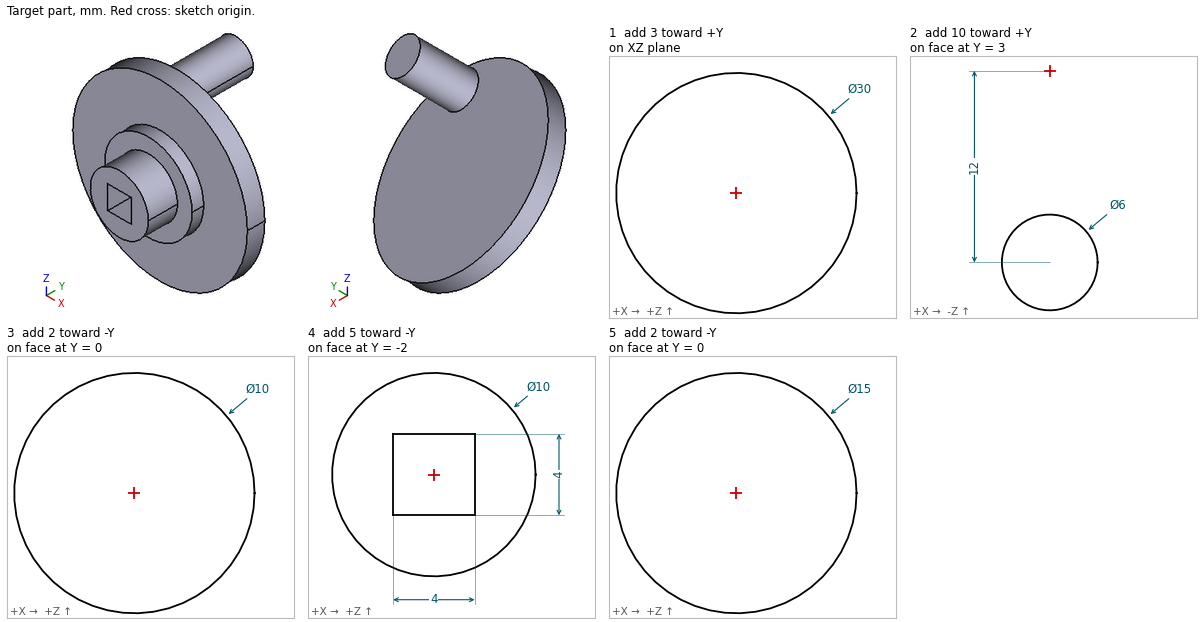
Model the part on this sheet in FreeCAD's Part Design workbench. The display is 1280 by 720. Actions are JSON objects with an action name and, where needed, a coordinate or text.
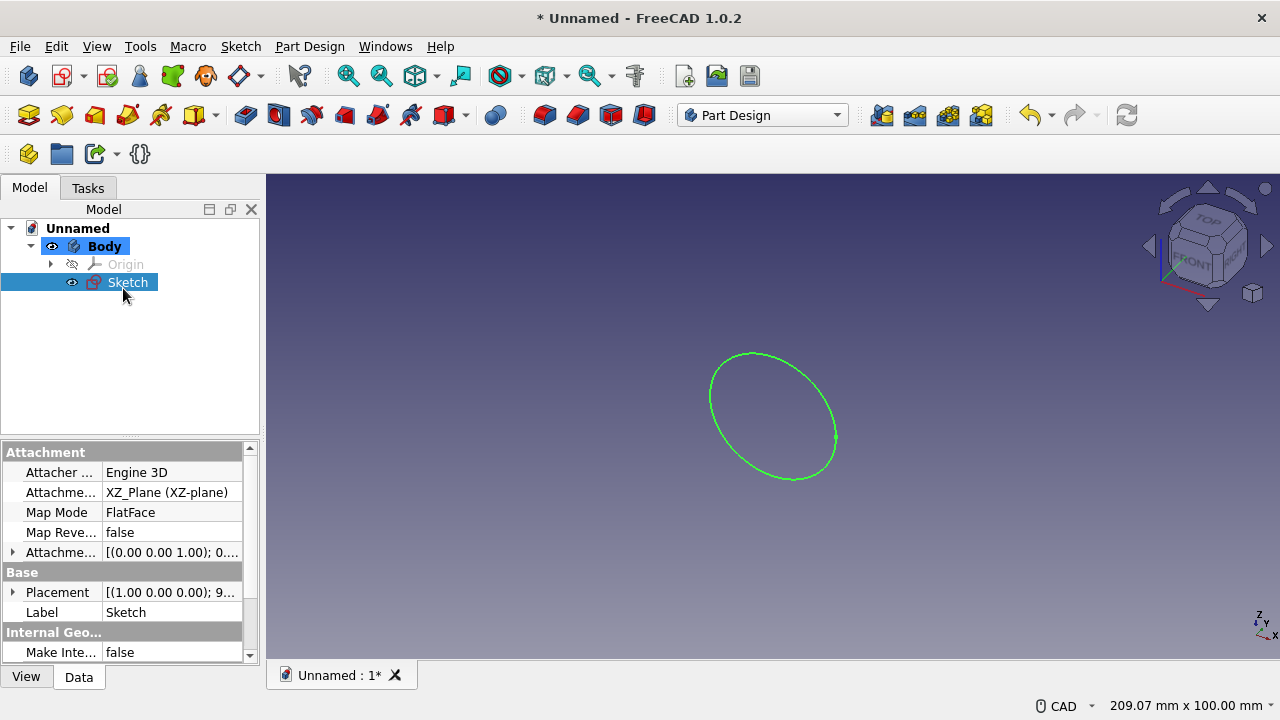
{"action": "left_click", "coordinate": [29, 116]}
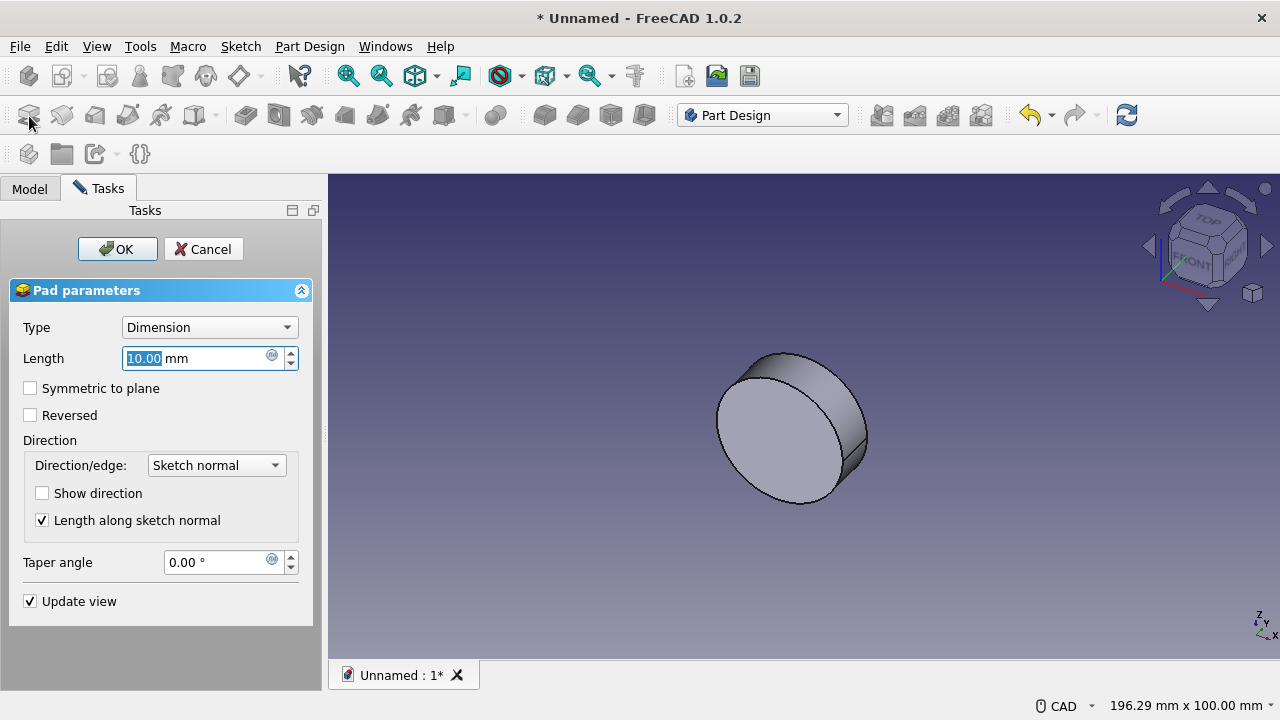
{"action": "type", "text": "3"}
{"action": "key", "text": "Tab"}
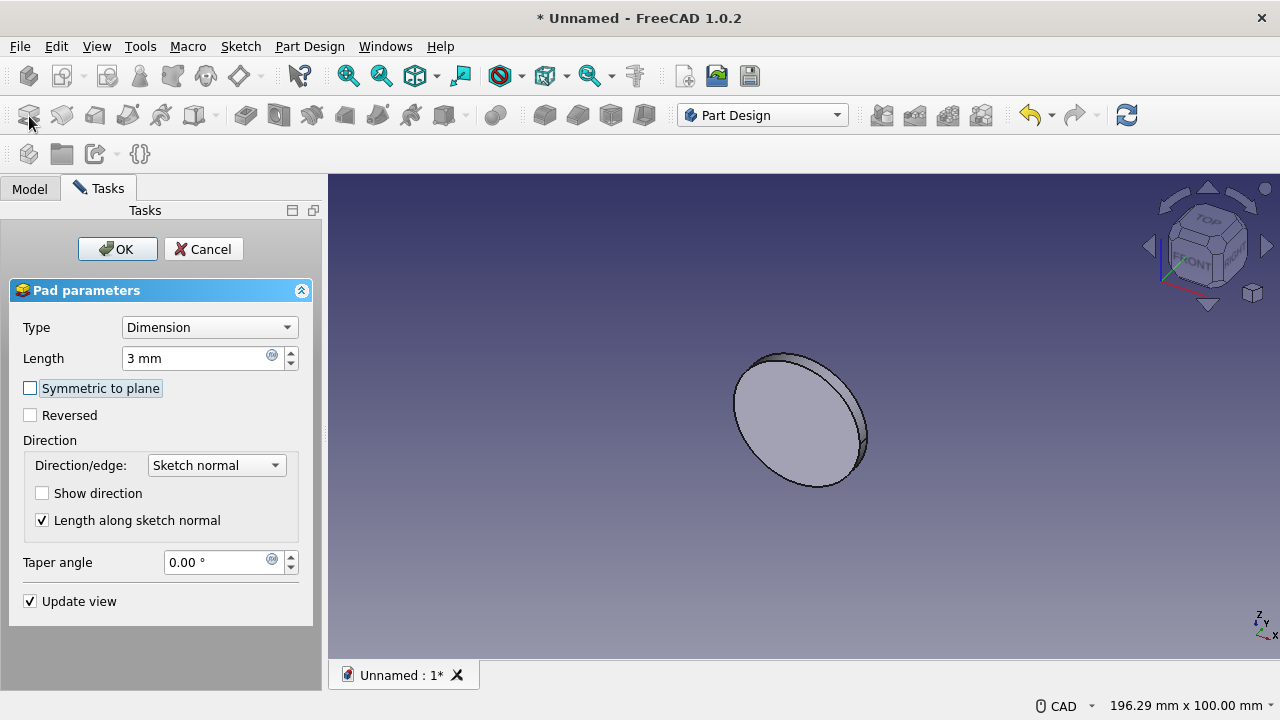
{"action": "left_click", "coordinate": [31, 415]}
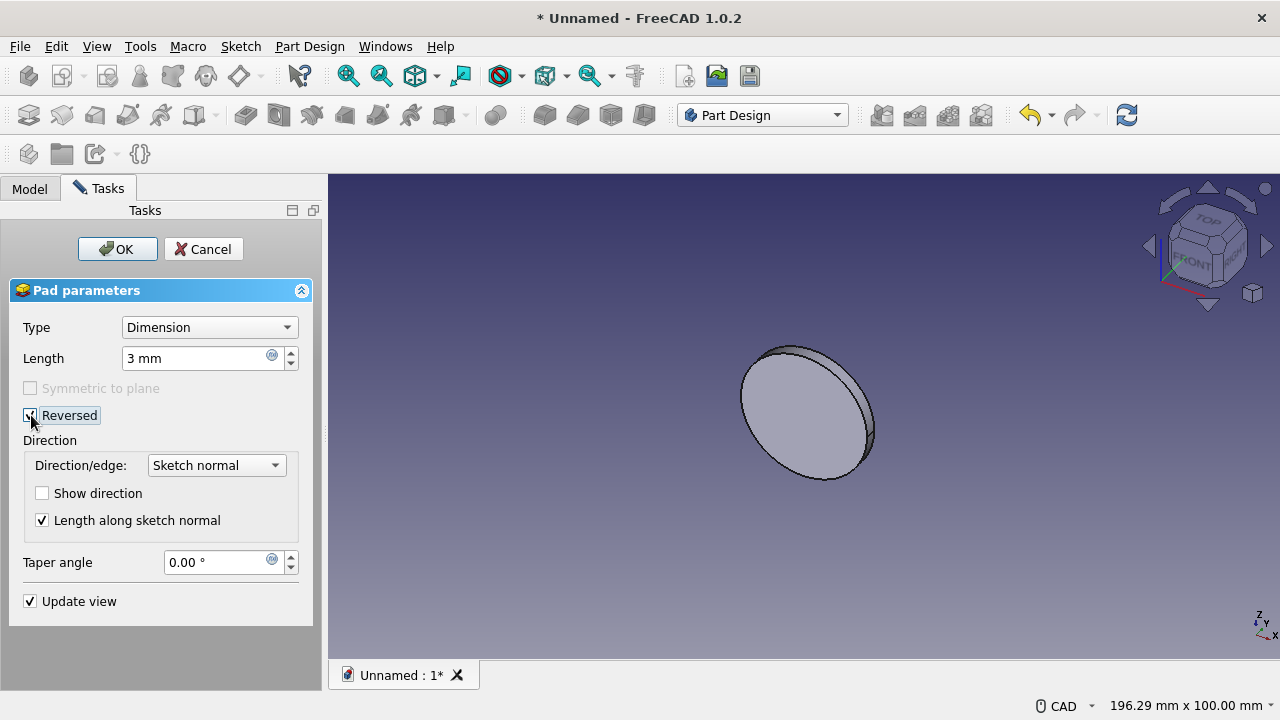
{"action": "left_click", "coordinate": [118, 249]}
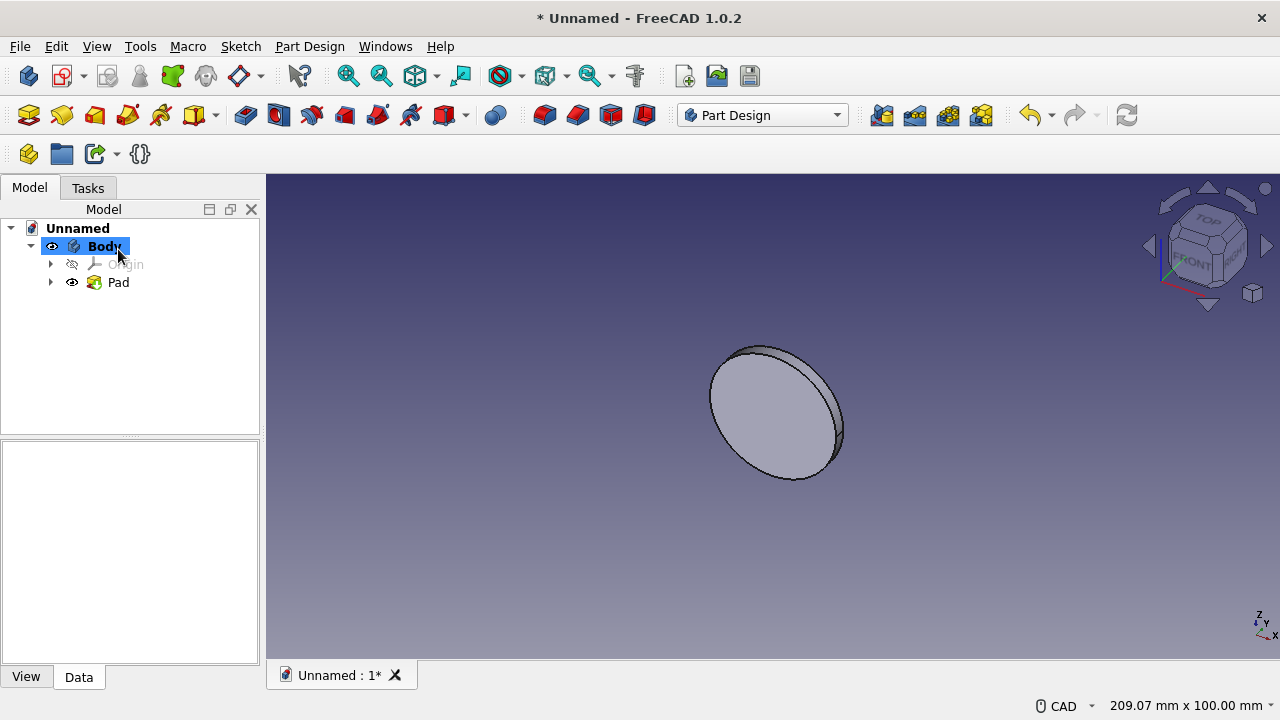
{"action": "left_click", "coordinate": [349, 76]}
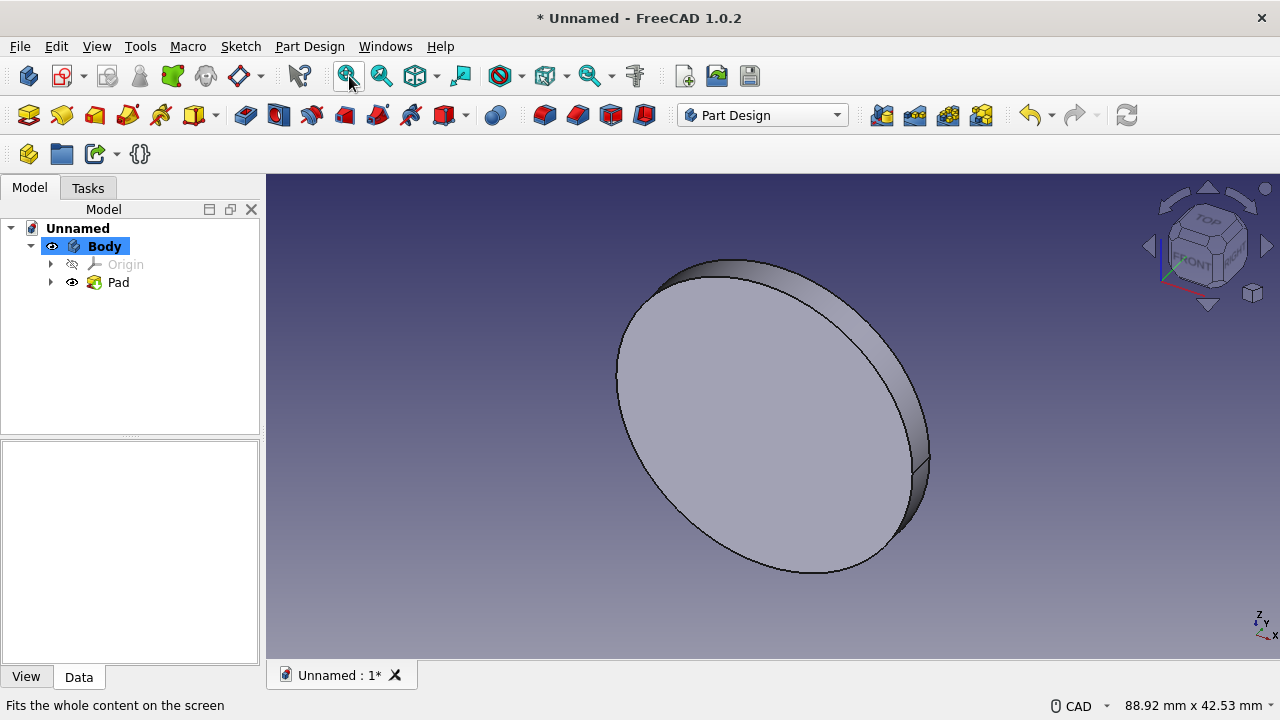
{"action": "key", "text": "4"}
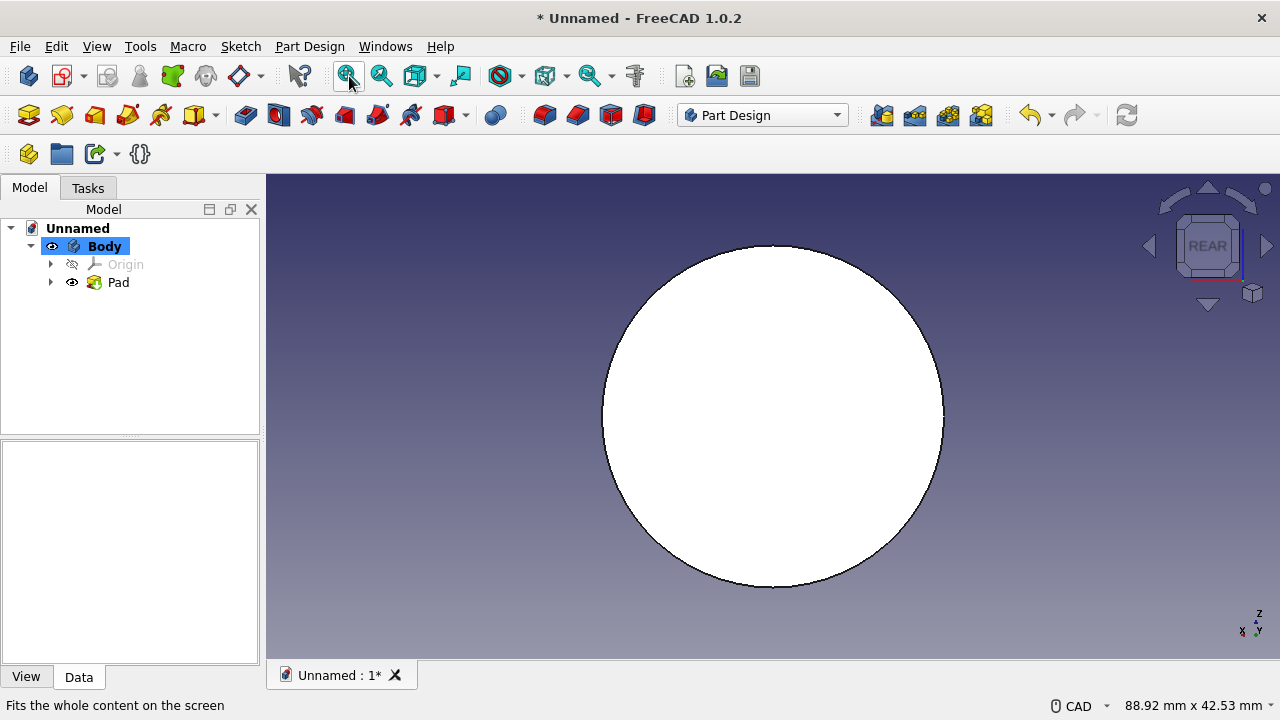
{"action": "left_click", "coordinate": [773, 415]}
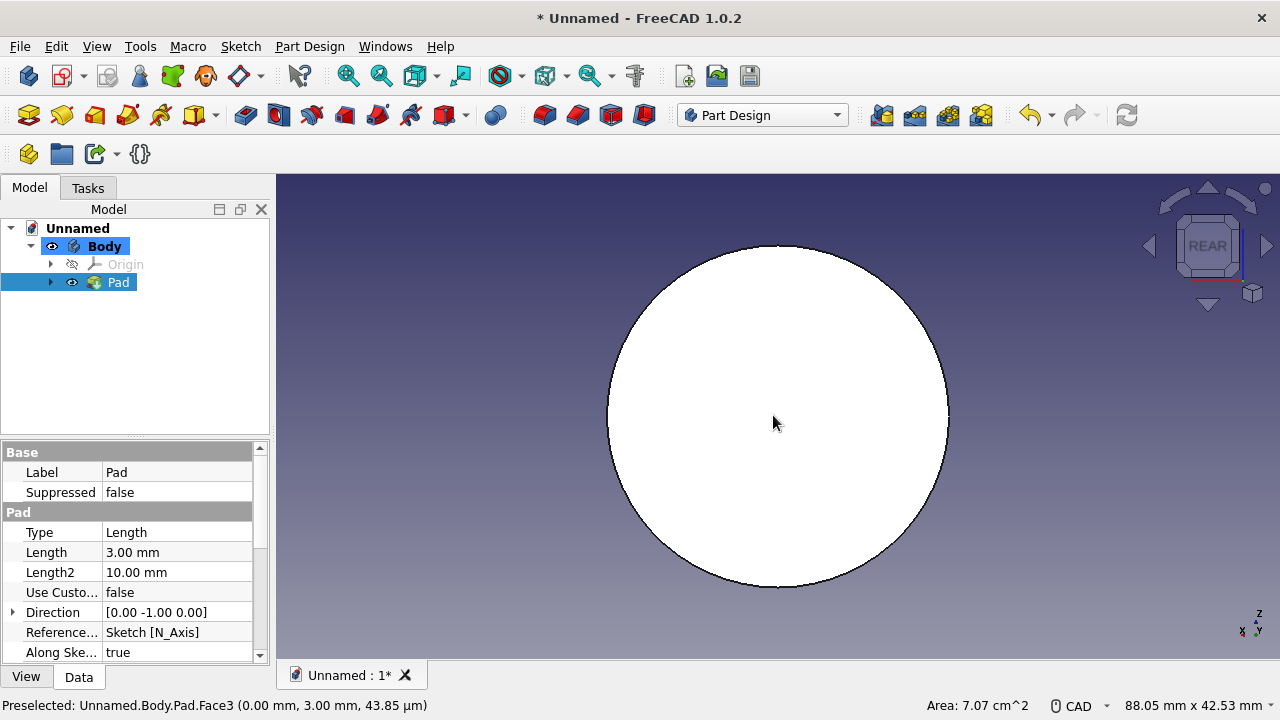
{"action": "left_click", "coordinate": [62, 76]}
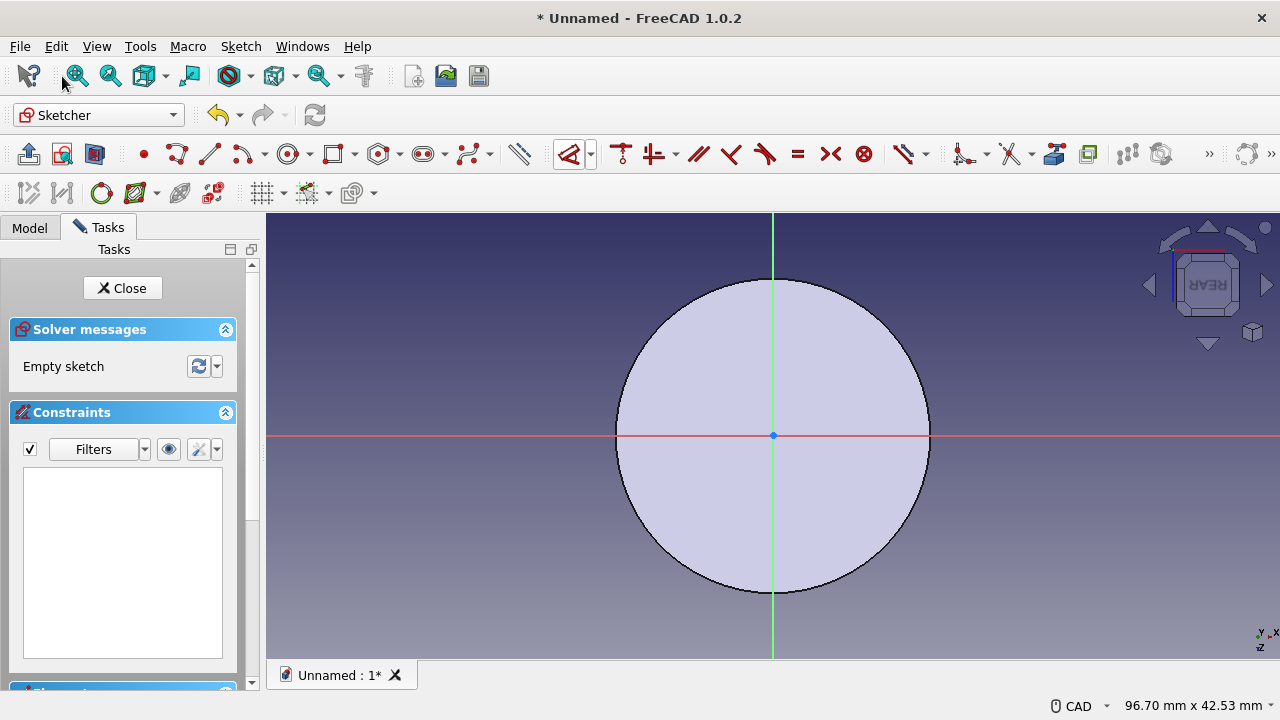
{"action": "scroll", "coordinate": [795, 603], "scroll_direction": "up", "scroll_amount": 7}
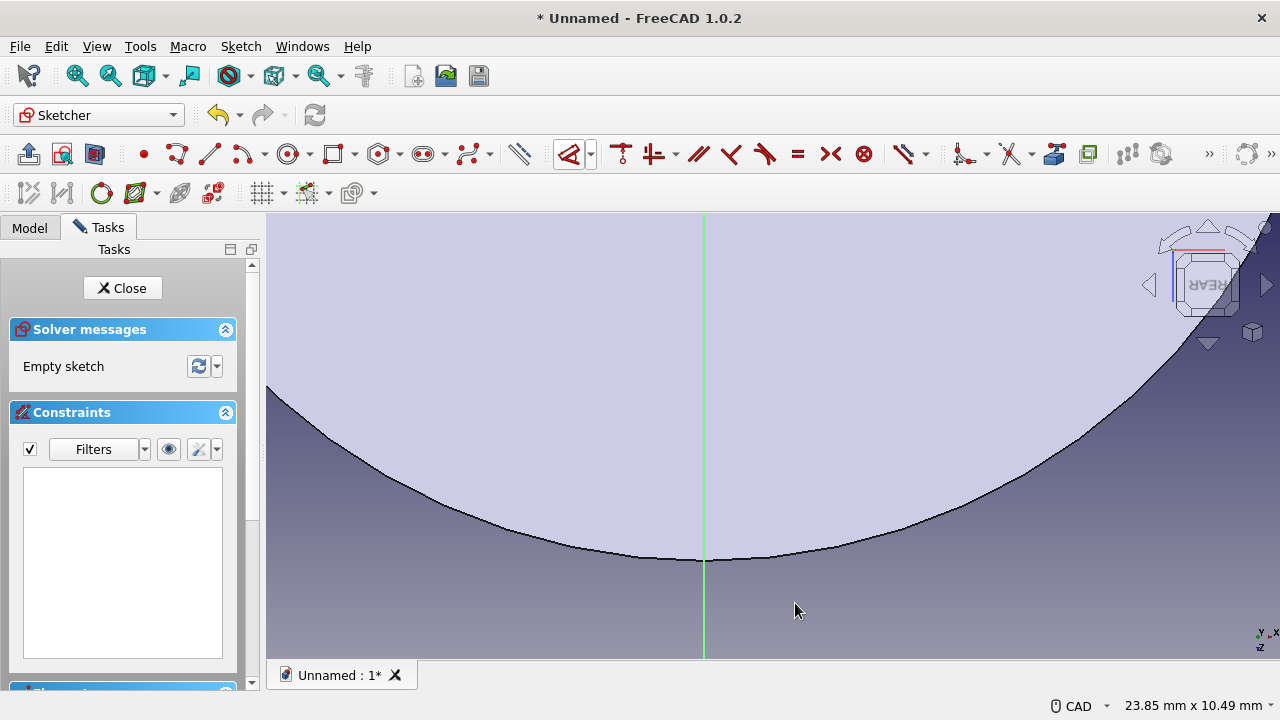
{"action": "key", "text": "g c"}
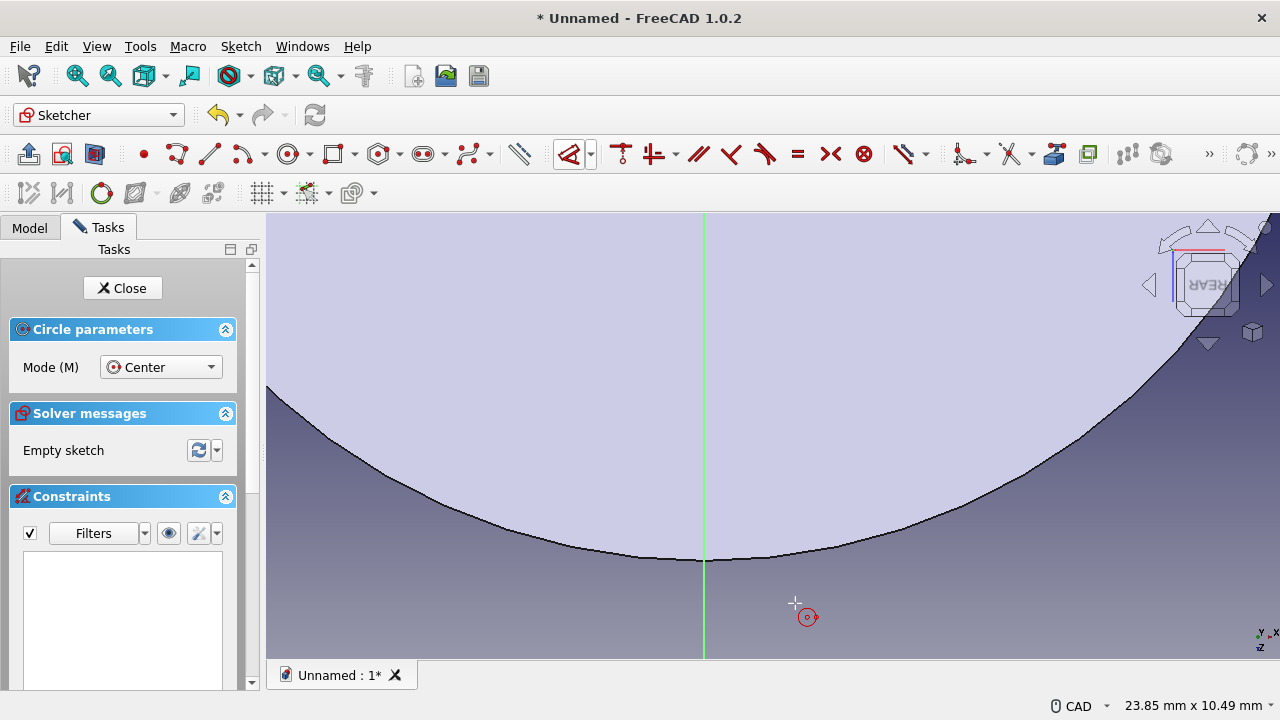
{"action": "left_click", "coordinate": [704, 433]}
{"action": "left_click", "coordinate": [794, 343]}
{"action": "key", "text": "Escape"}